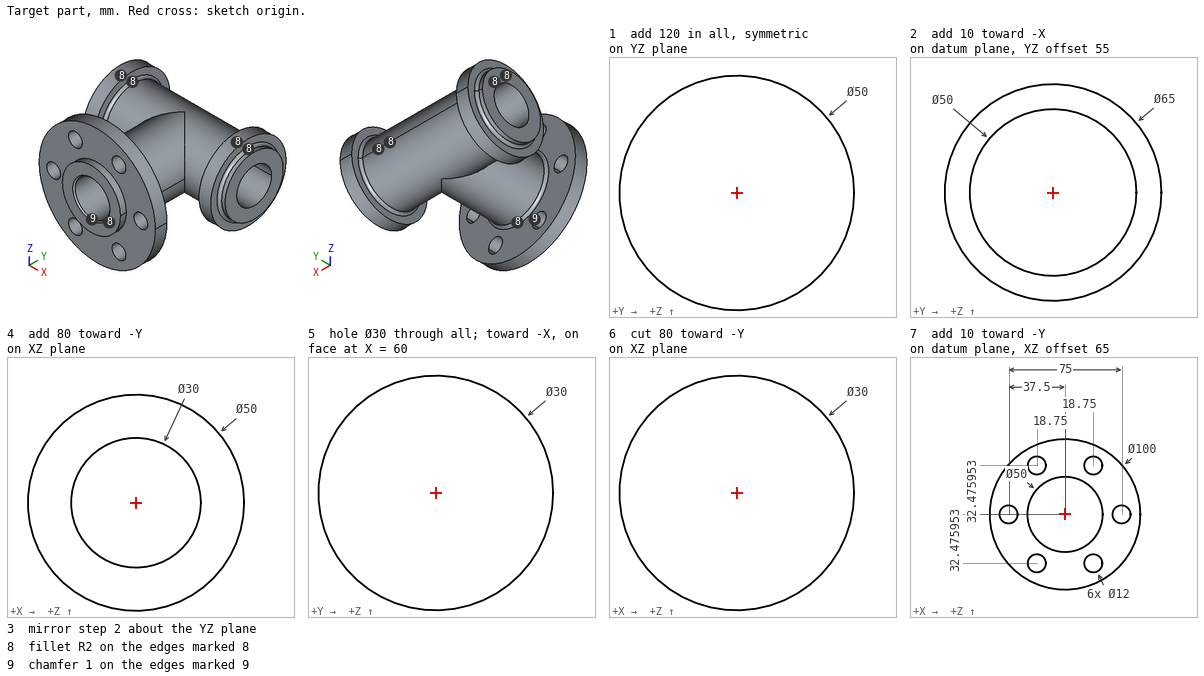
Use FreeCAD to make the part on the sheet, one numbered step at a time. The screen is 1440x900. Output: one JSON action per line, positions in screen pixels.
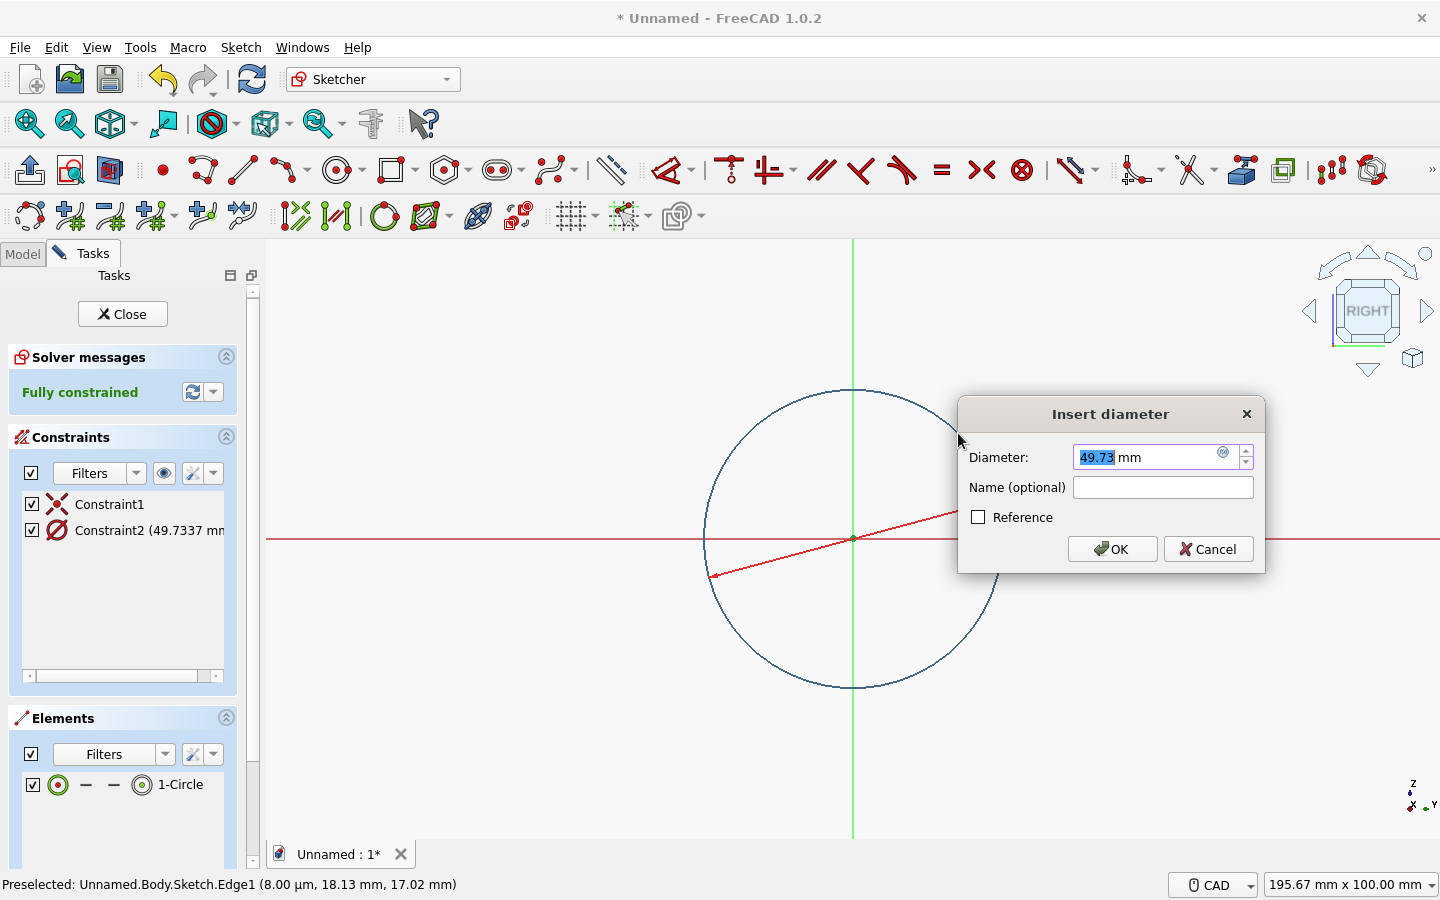
{"action": "type", "text": "50"}
{"action": "key", "text": "Return"}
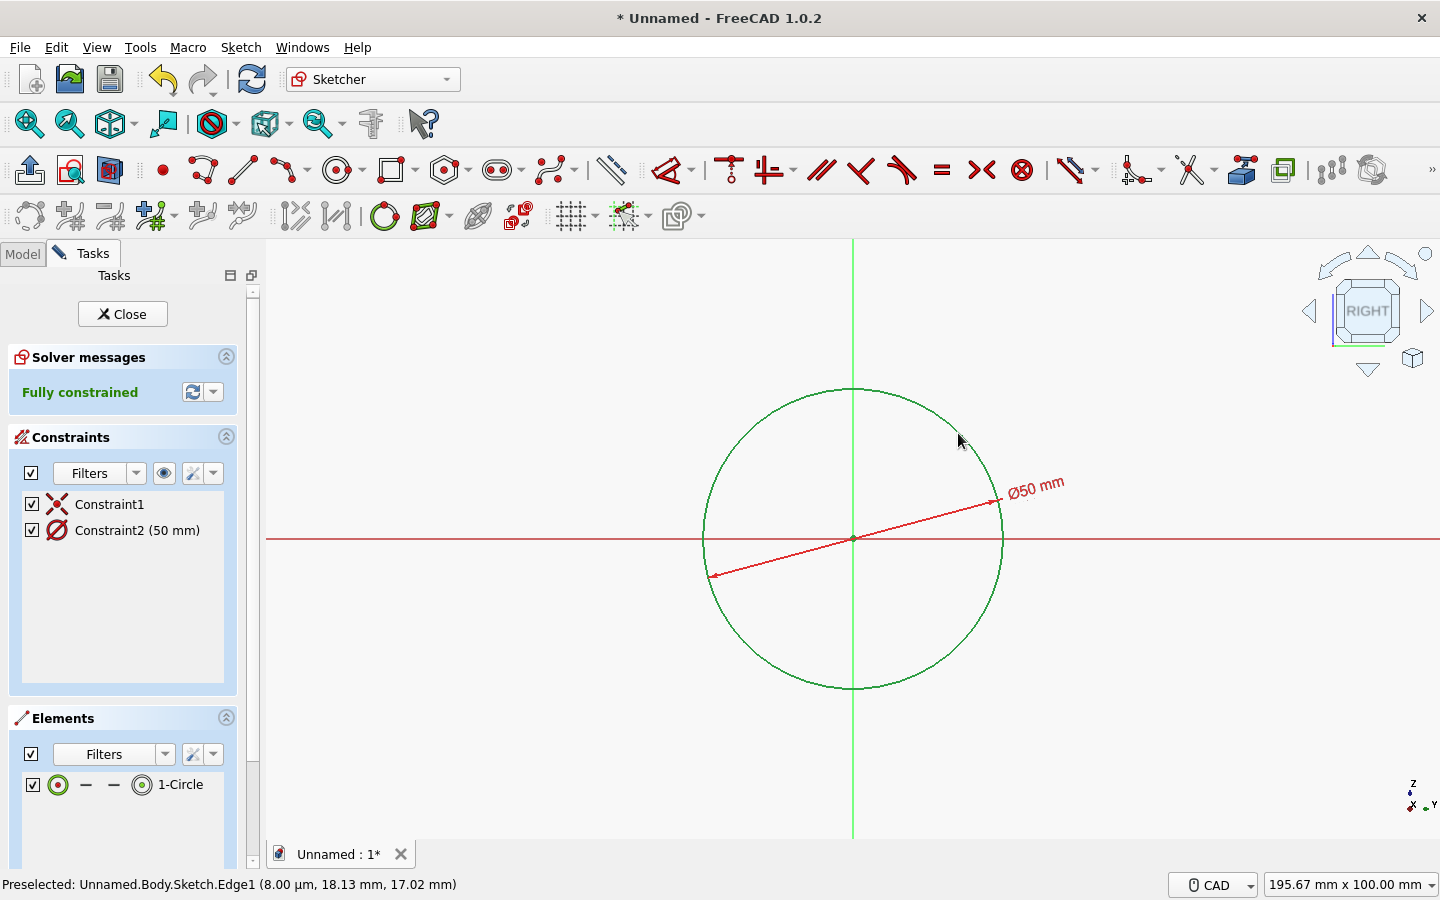
{"action": "left_click", "coordinate": [123, 314]}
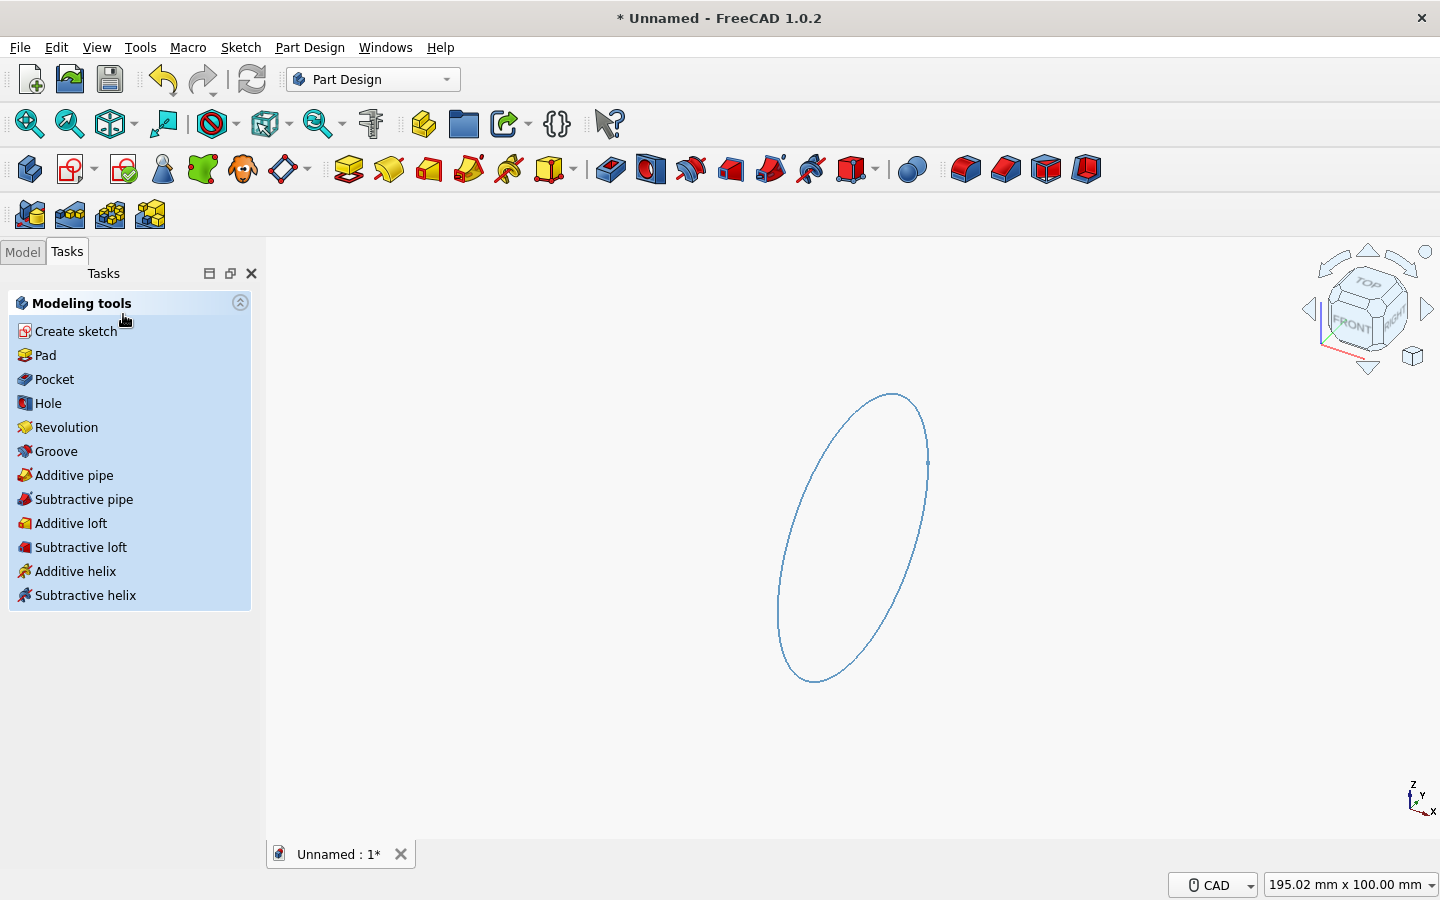
{"action": "left_click", "coordinate": [350, 170]}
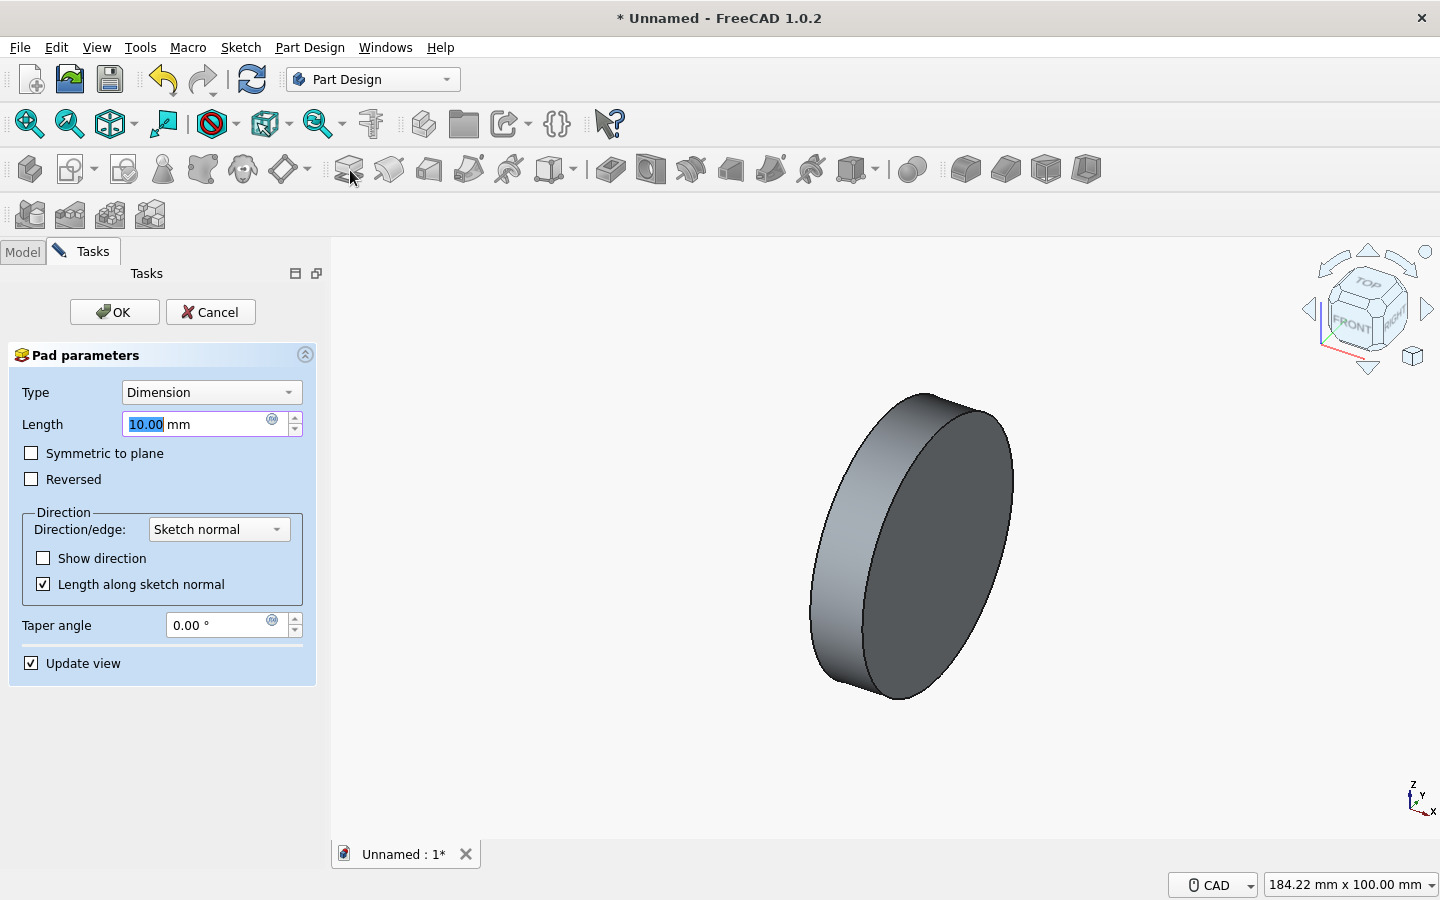
{"action": "type", "text": "120"}
{"action": "key", "text": "Tab"}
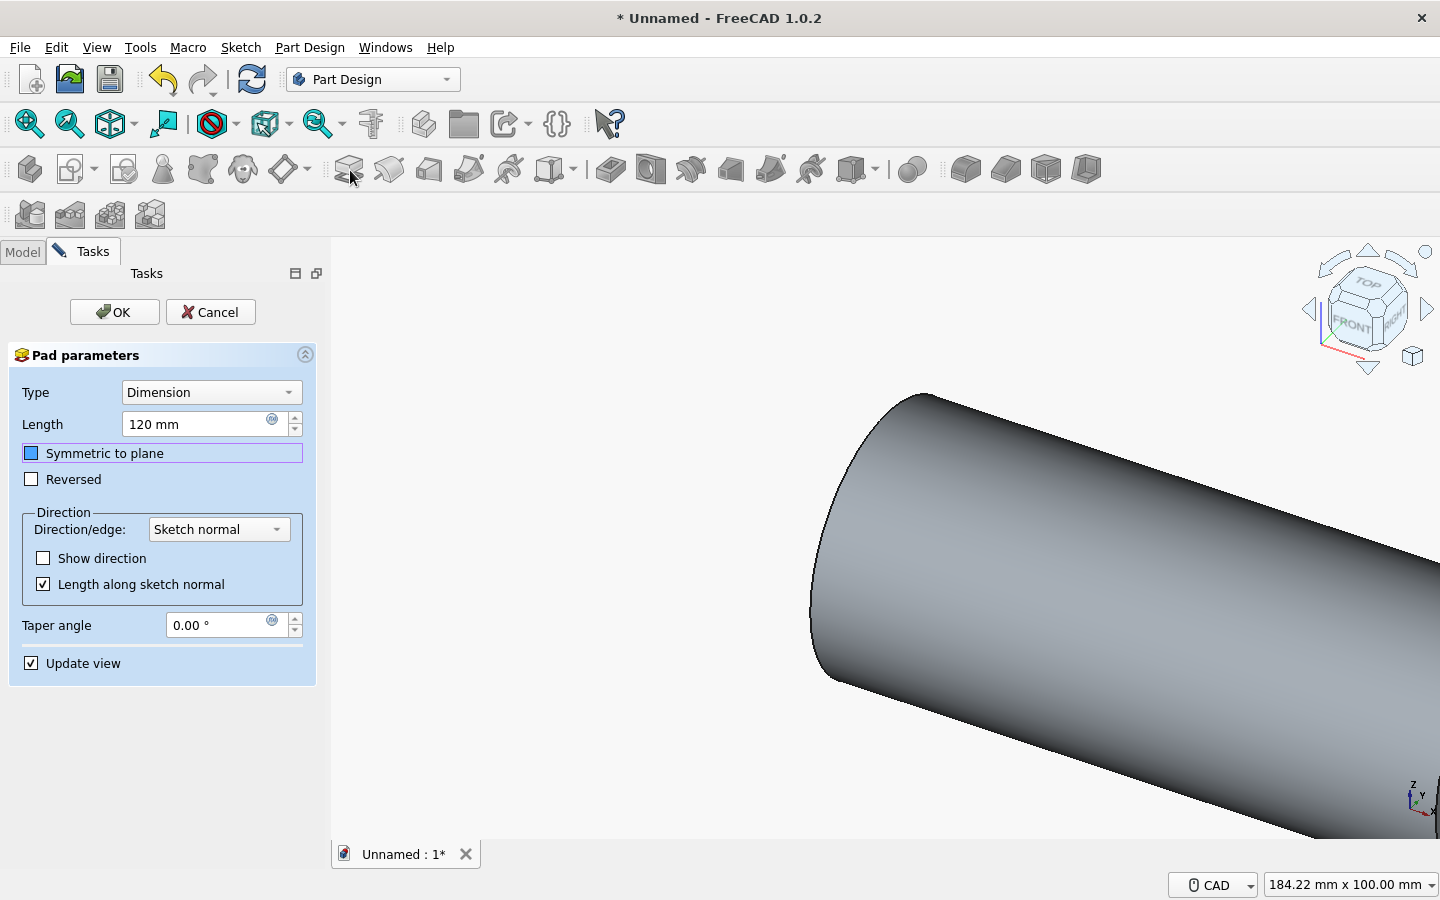
{"action": "left_click", "coordinate": [30, 453]}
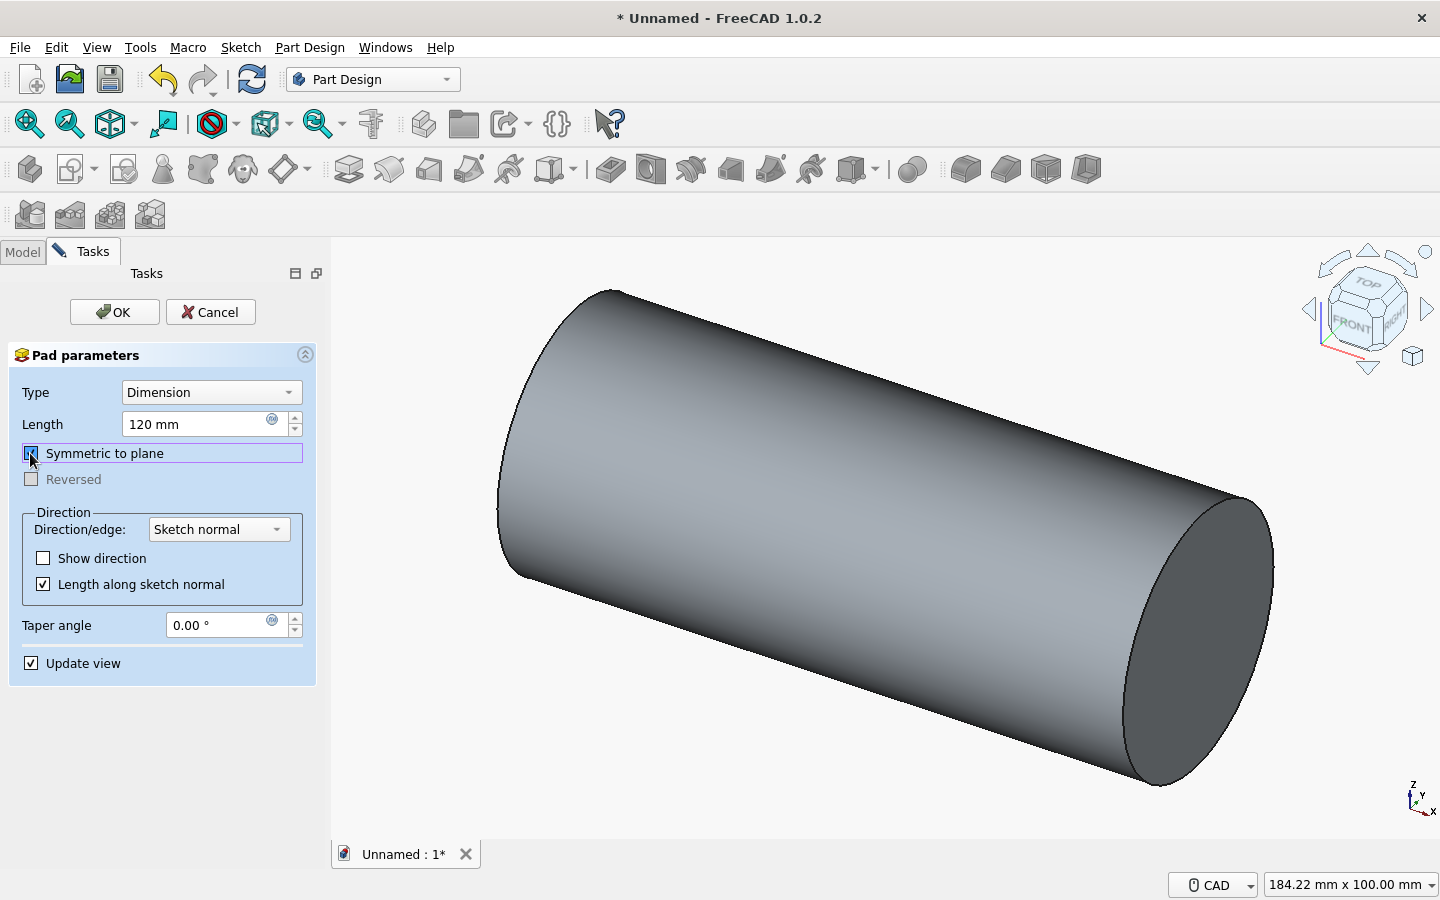
{"action": "left_click", "coordinate": [115, 312]}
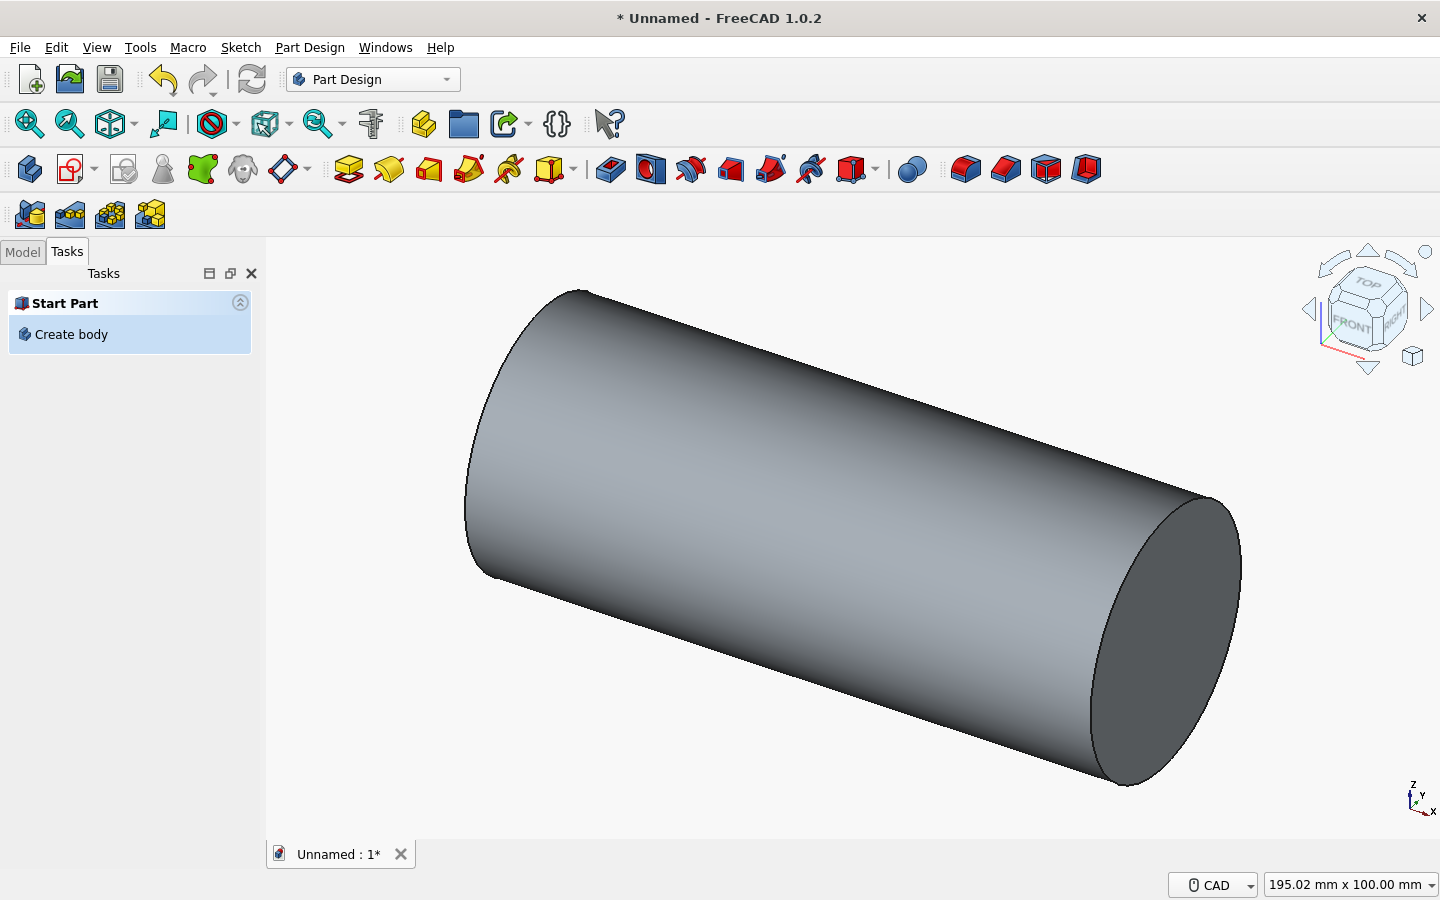
{"action": "key", "text": "v f"}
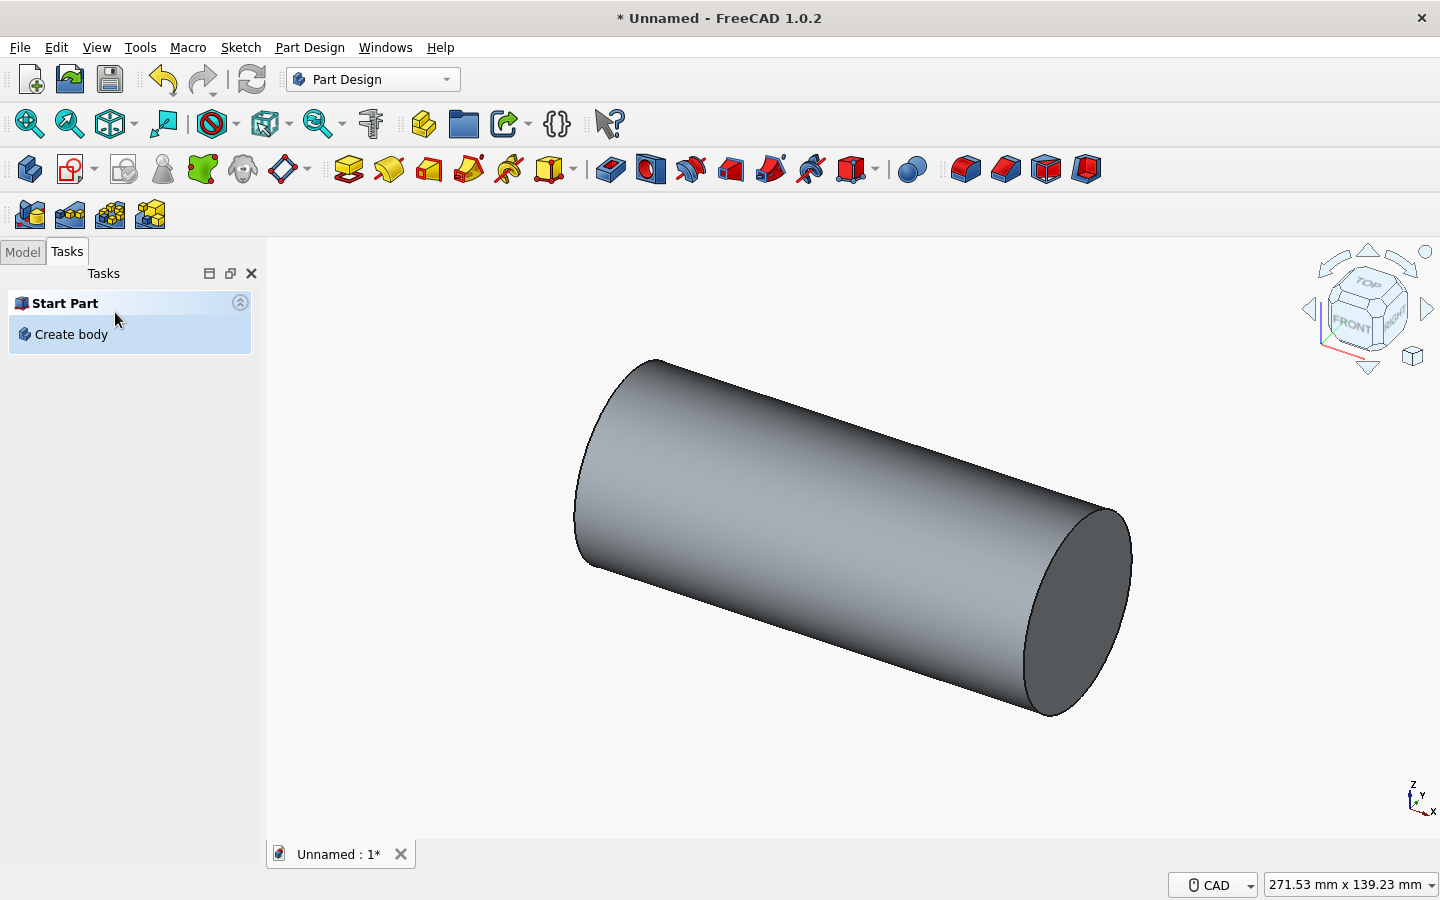
{"action": "left_click", "coordinate": [23, 251]}